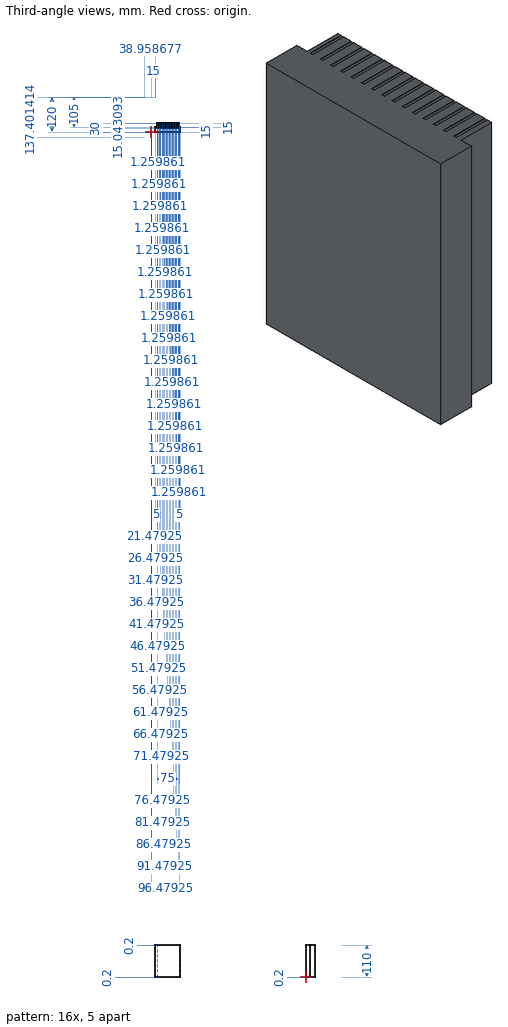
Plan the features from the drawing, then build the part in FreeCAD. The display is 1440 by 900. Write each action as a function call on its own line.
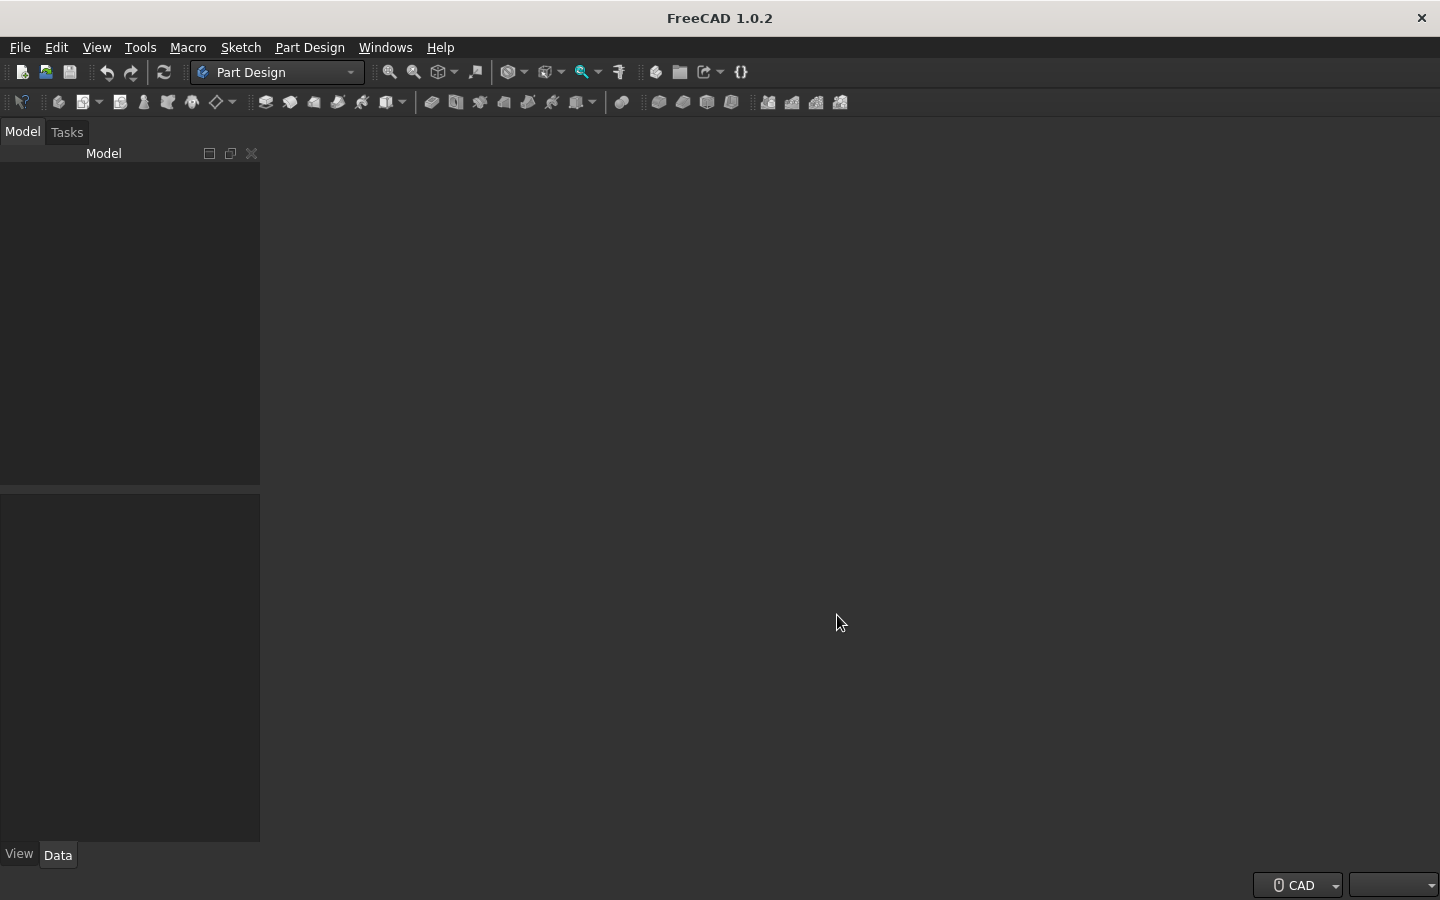
click(22, 72)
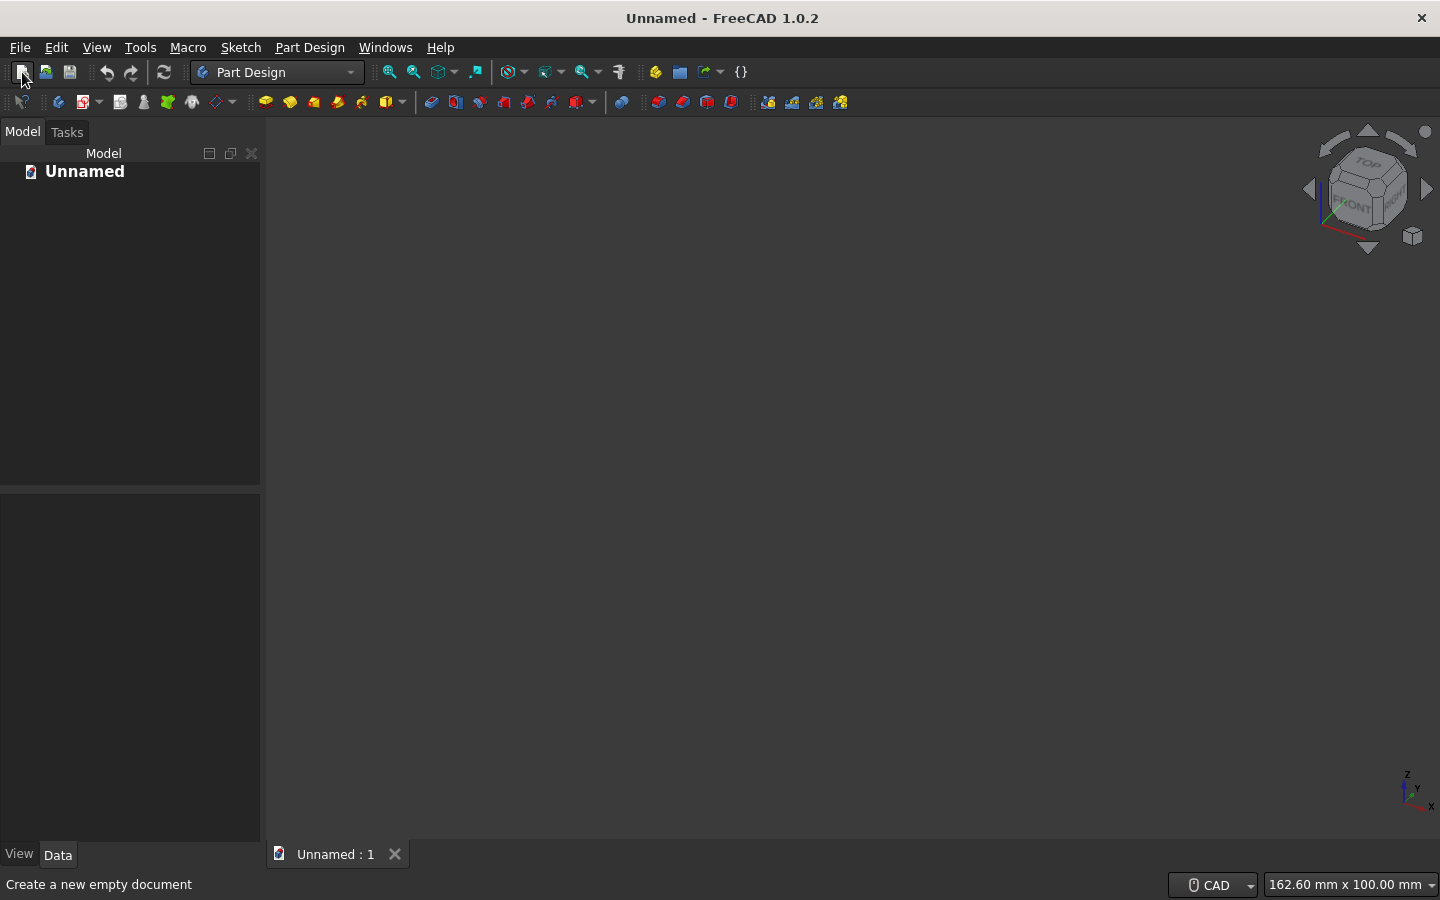
click(84, 102)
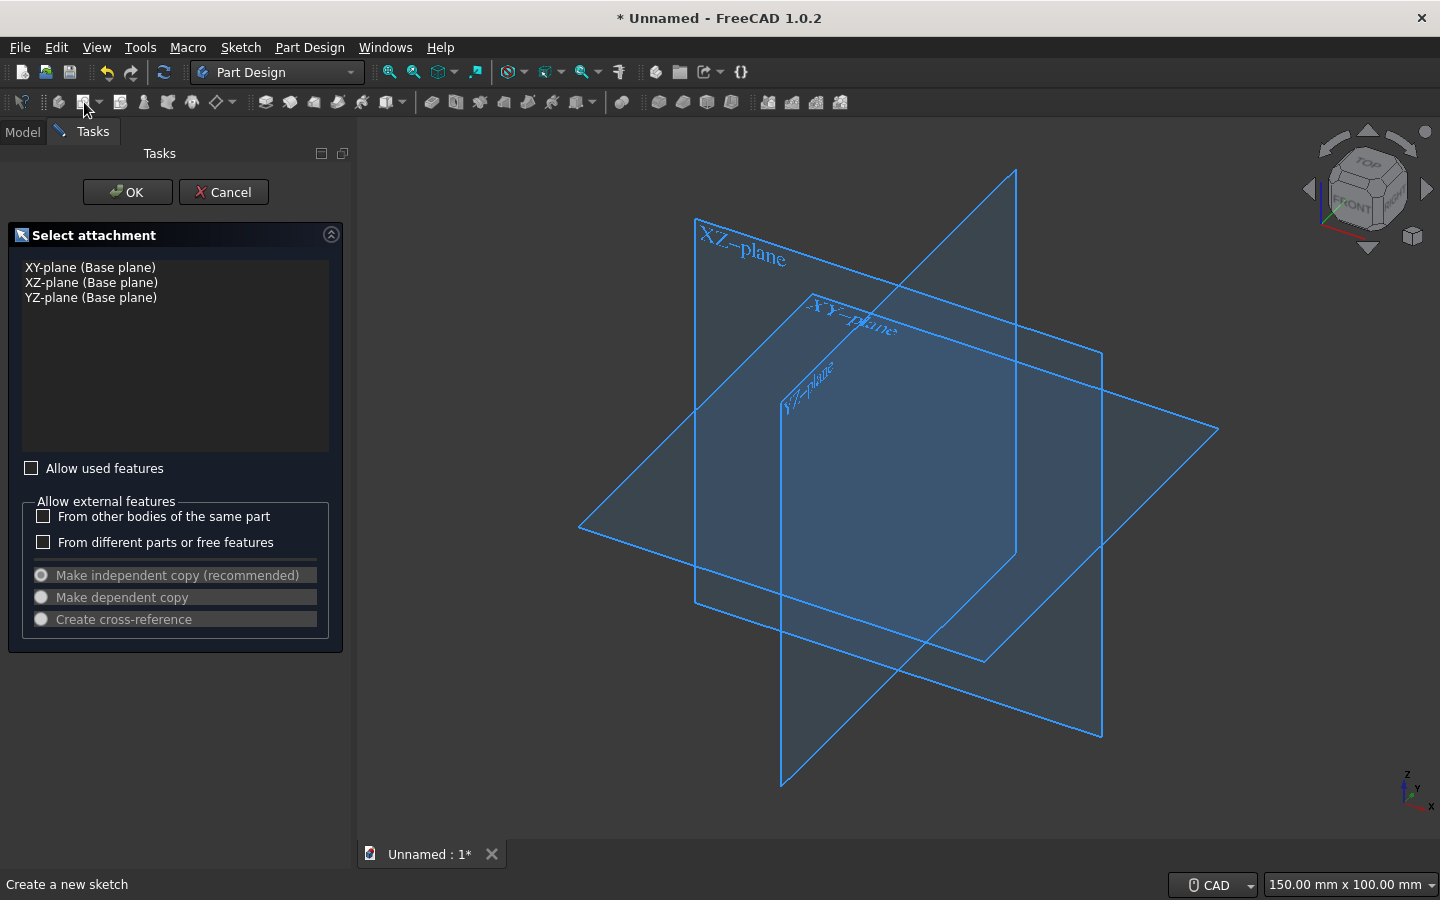
click(82, 268)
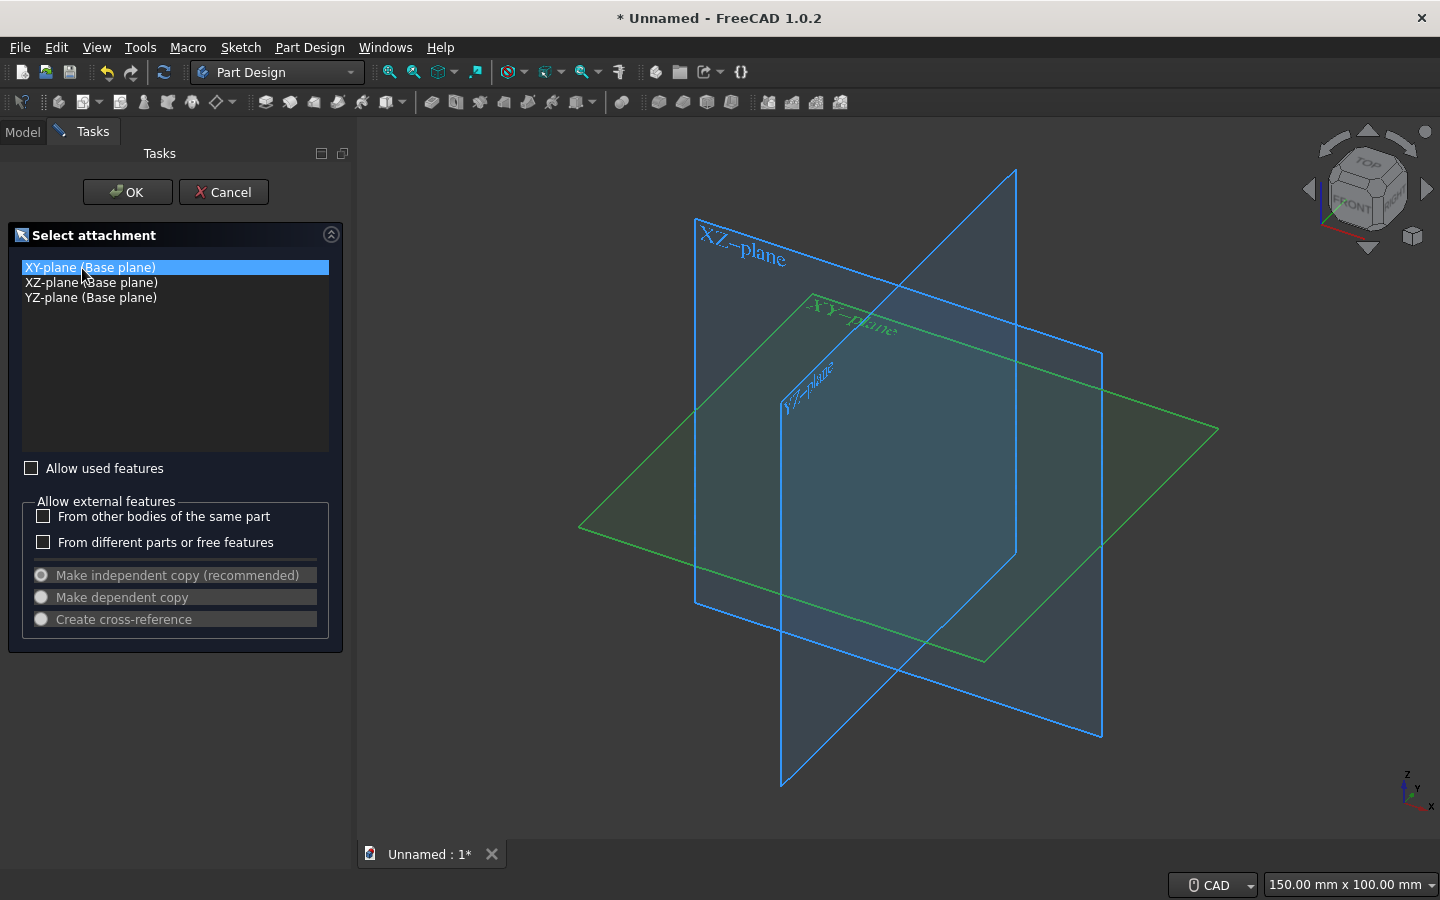
click(128, 192)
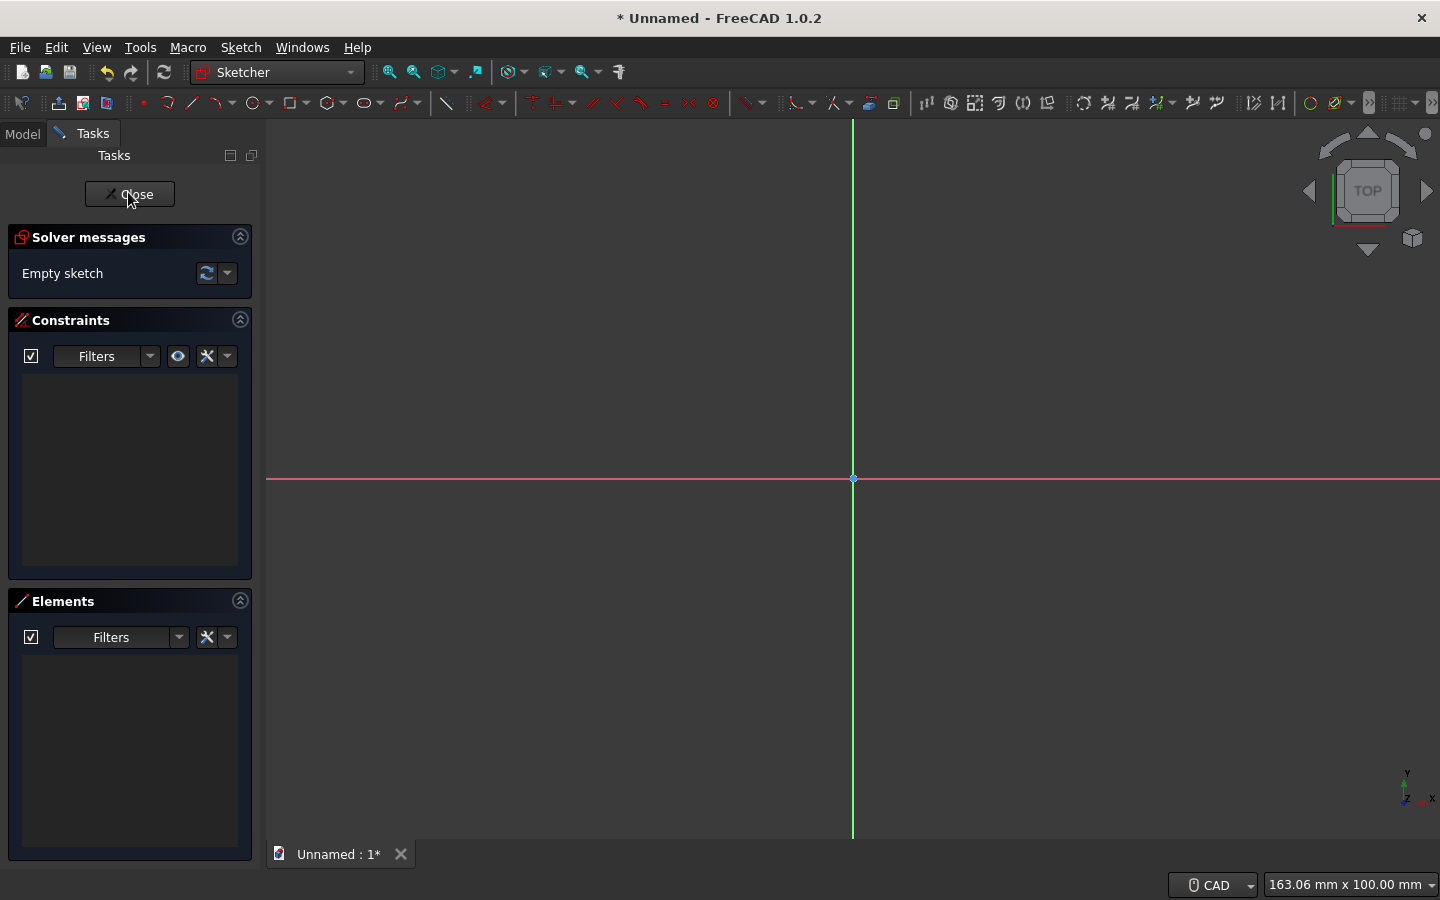
scroll(435, 811, down, 4)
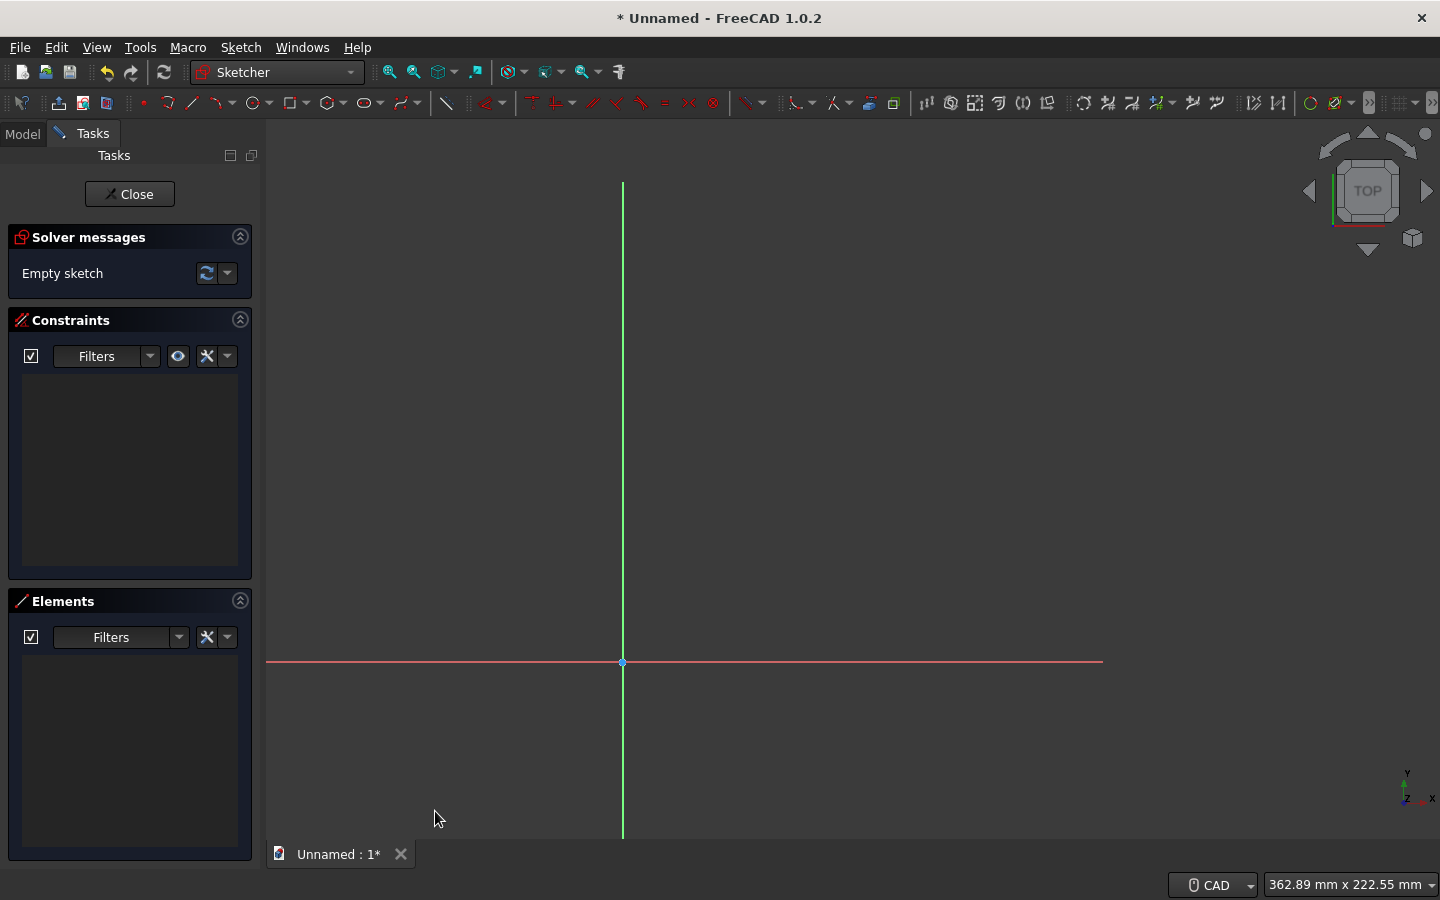
key(g)
key(m)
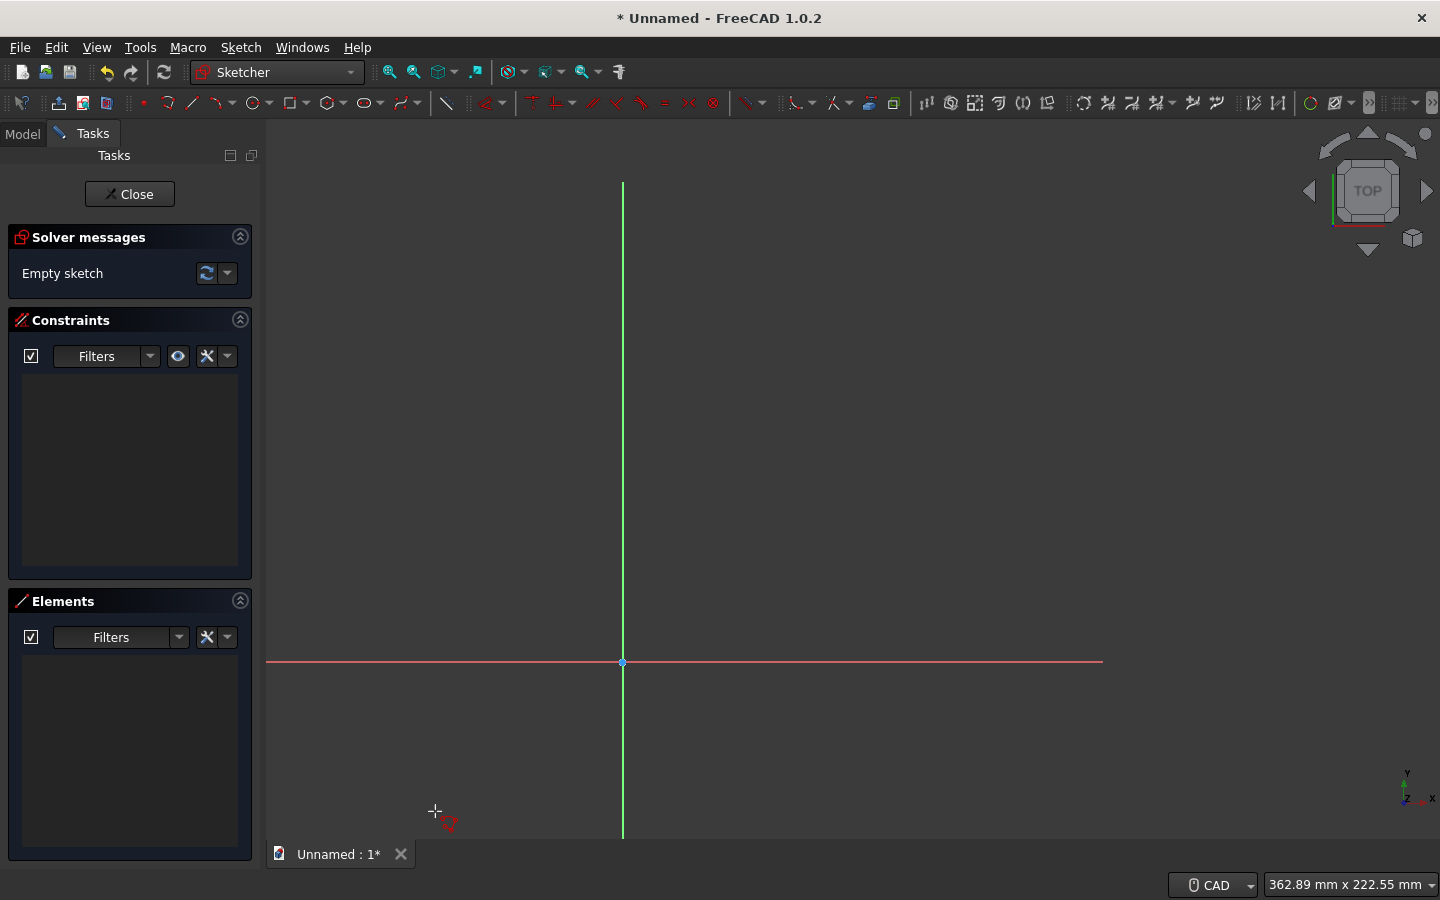
click(623, 662)
click(946, 653)
click(946, 614)
click(930, 614)
click(930, 565)
click(688, 565)
click(688, 614)
click(671, 614)
click(671, 274)
click(632, 274)
click(623, 662)
key(Escape)
key(Escape)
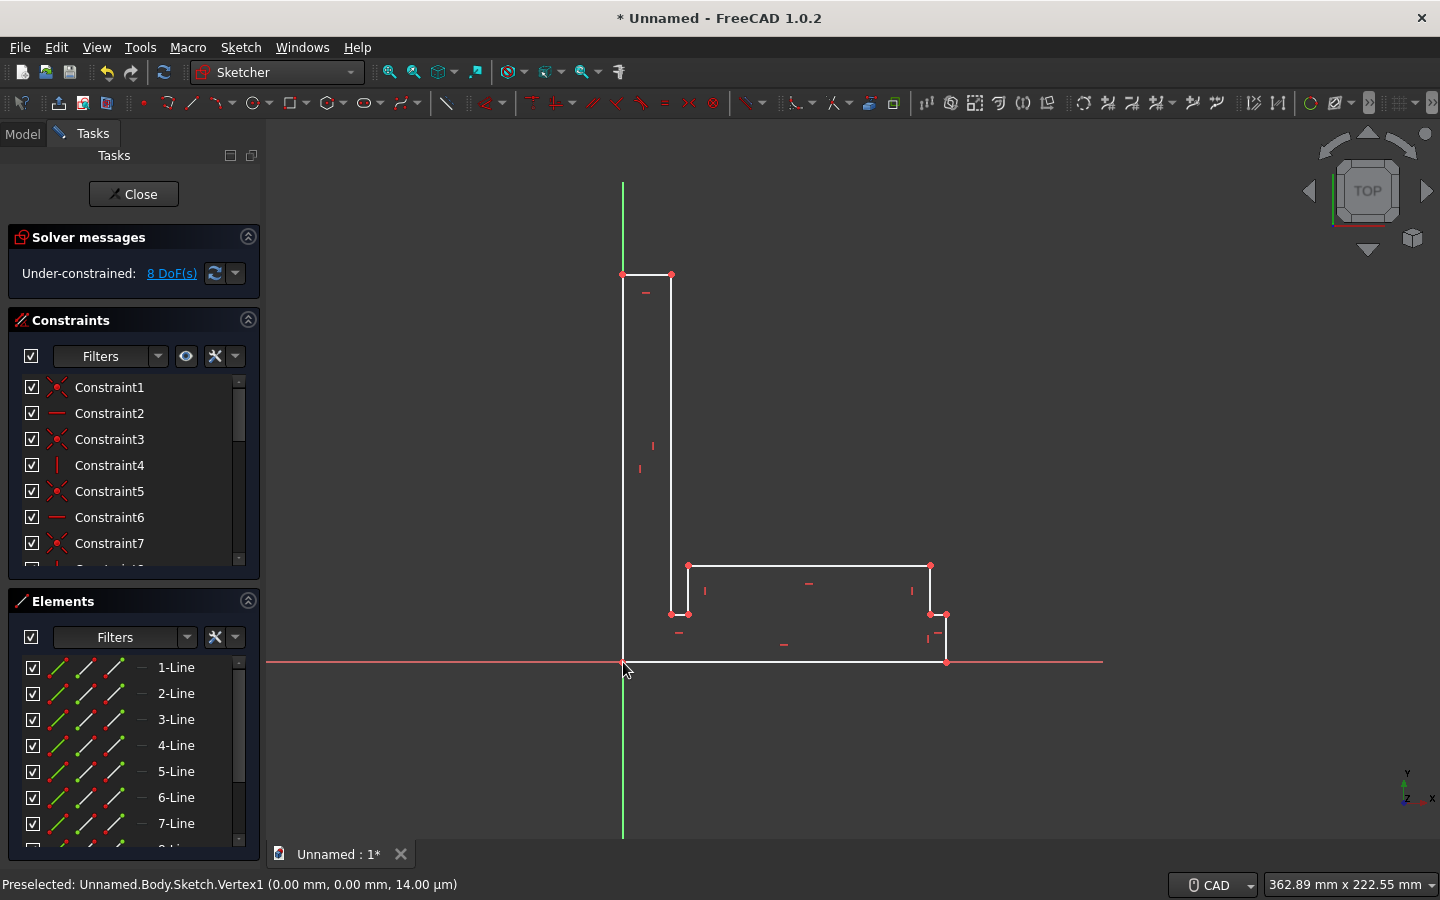
click(486, 104)